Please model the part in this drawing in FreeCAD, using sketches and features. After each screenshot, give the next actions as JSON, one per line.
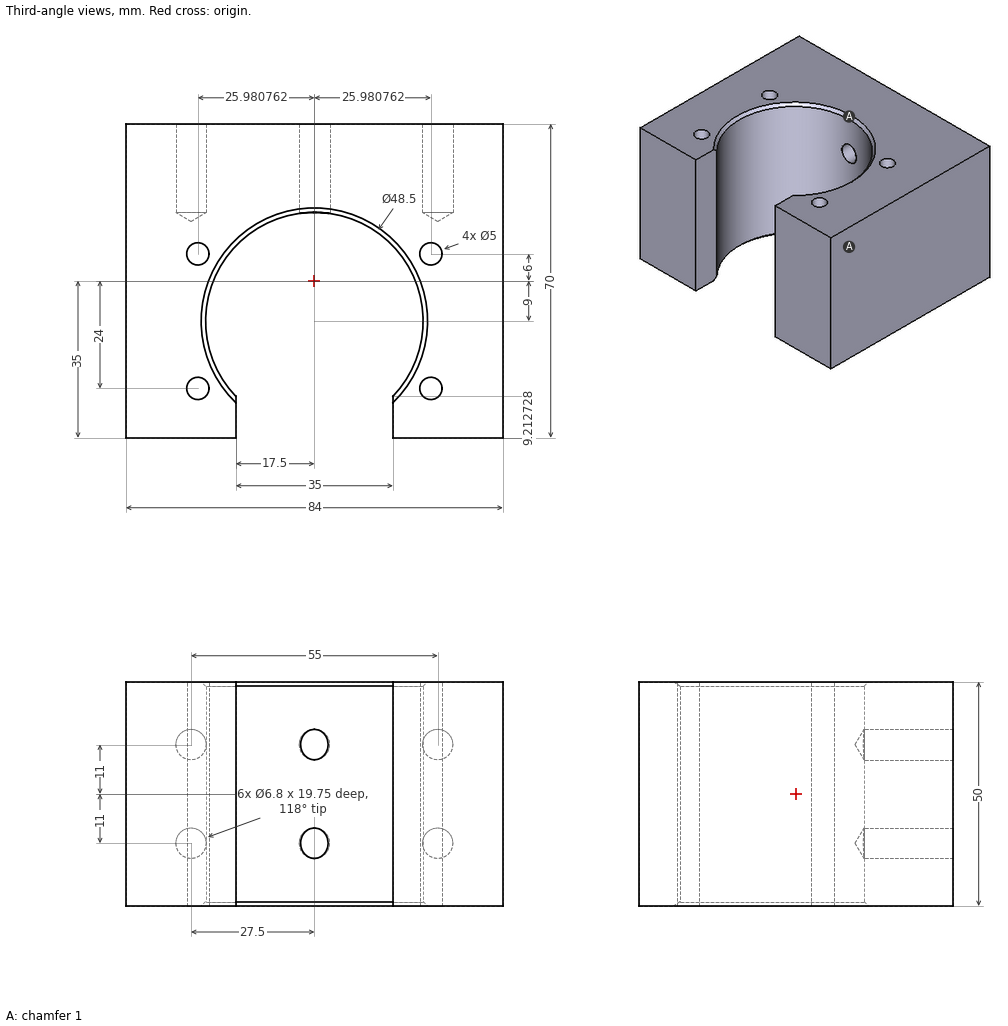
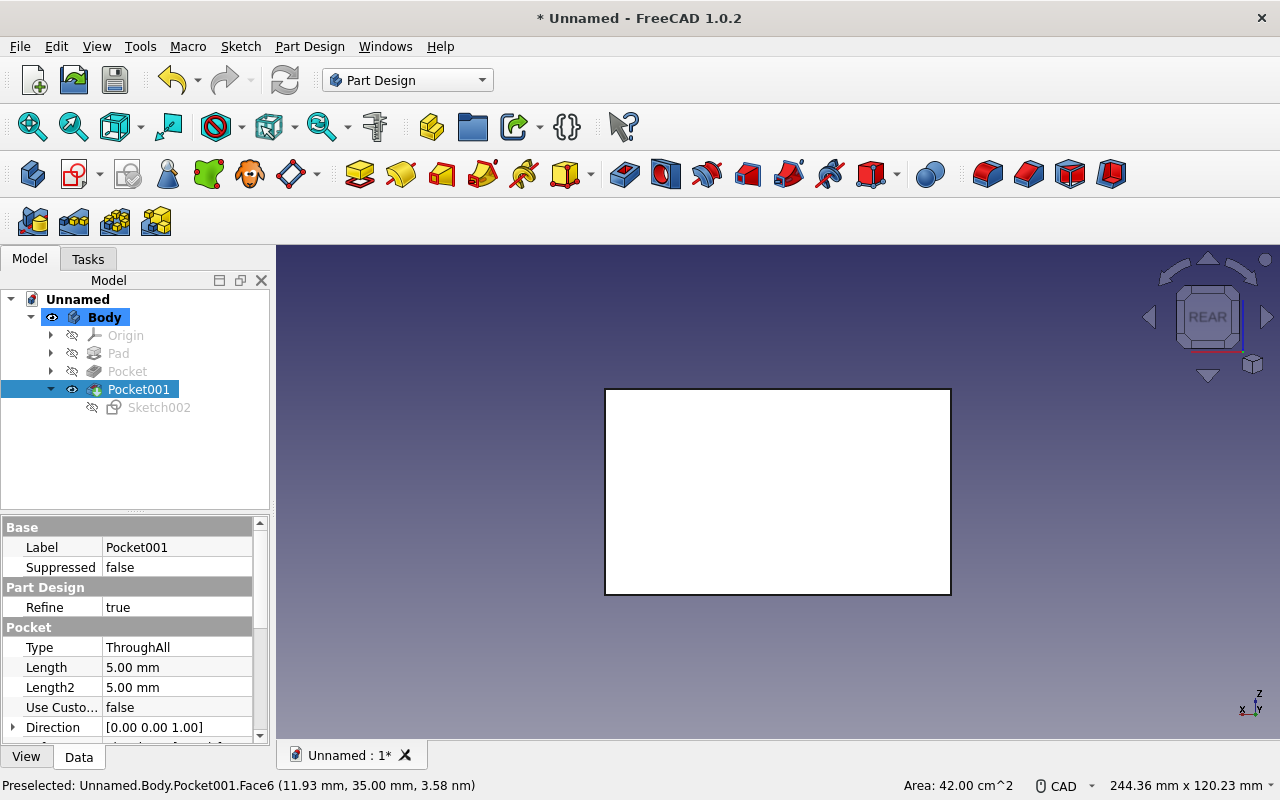
{"action": "left_click", "coordinate": [74, 174]}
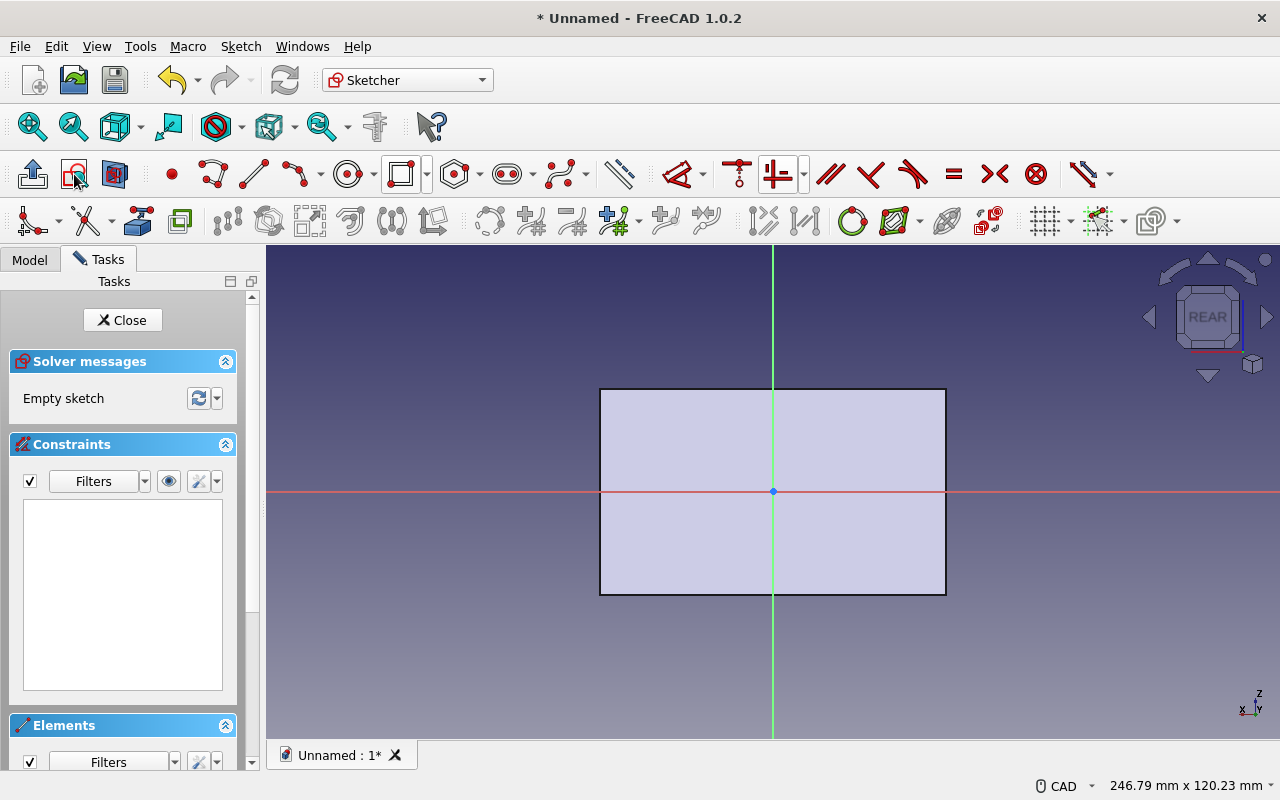
{"action": "scroll", "coordinate": [829, 492], "scroll_direction": "up", "scroll_amount": 4}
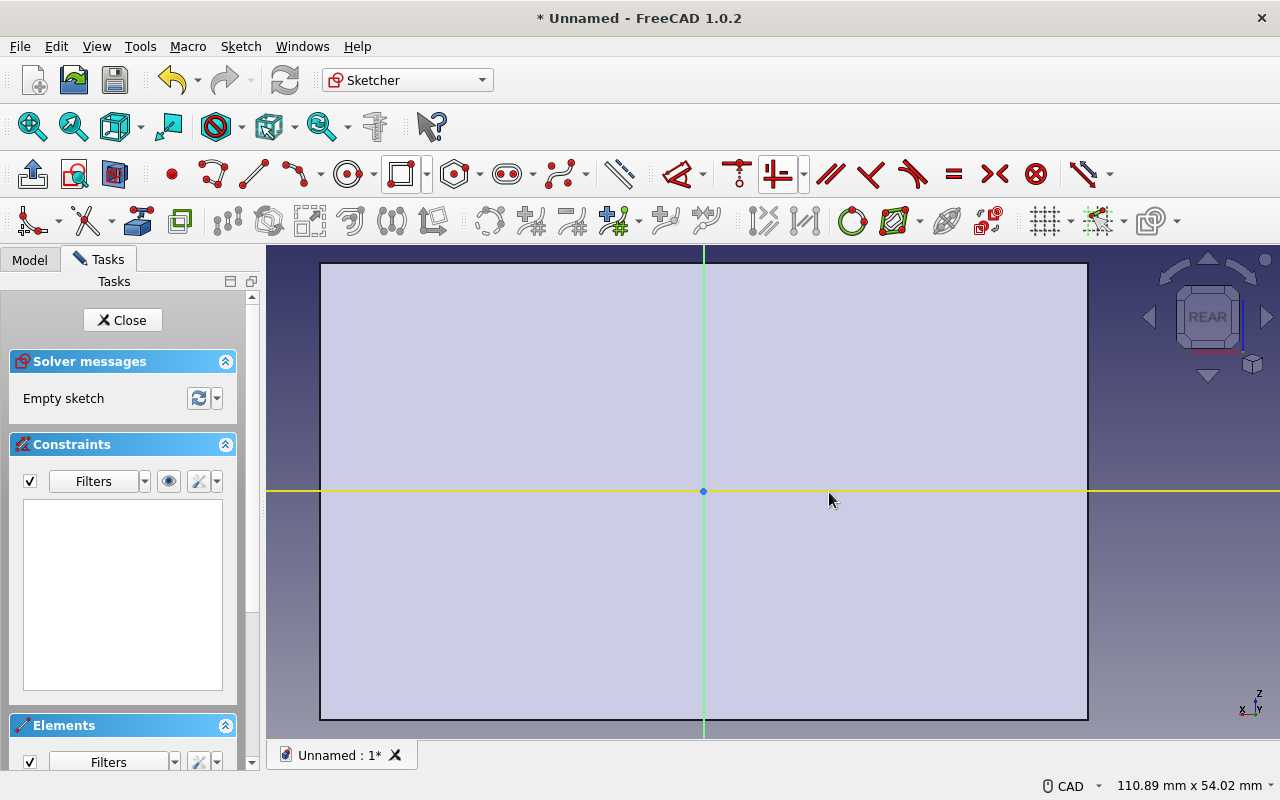
{"action": "left_click", "coordinate": [348, 174]}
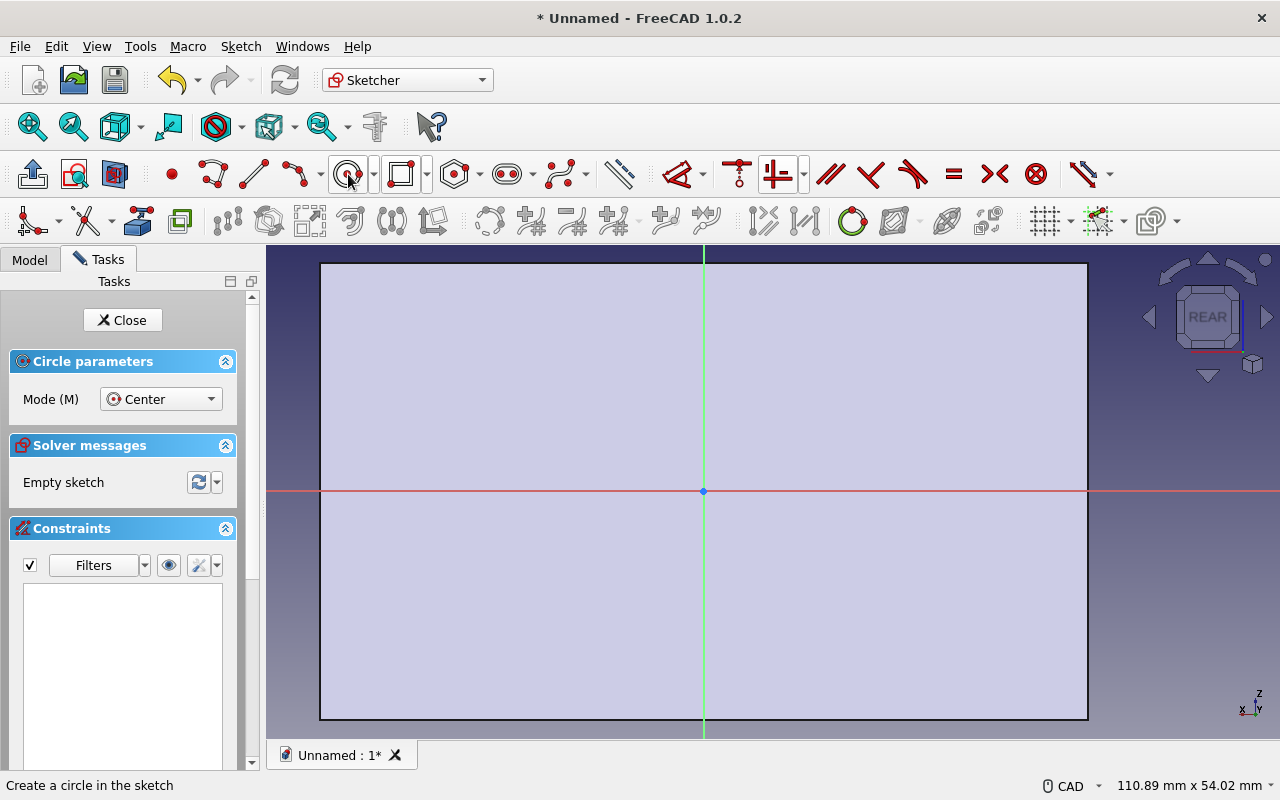
{"action": "left_click", "coordinate": [955, 592]}
{"action": "mouse_move", "coordinate": [977, 570]}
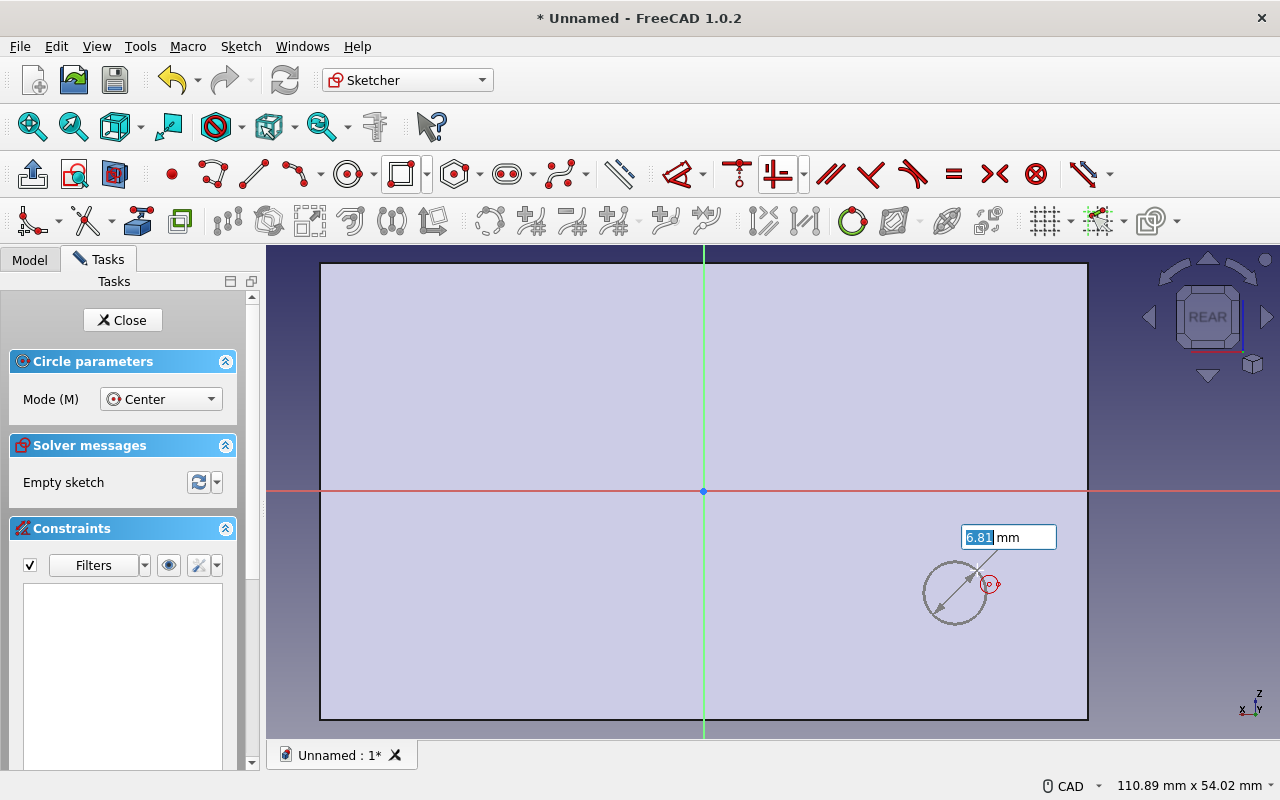
{"action": "type", "text": "6.8"}
{"action": "key", "text": "Return"}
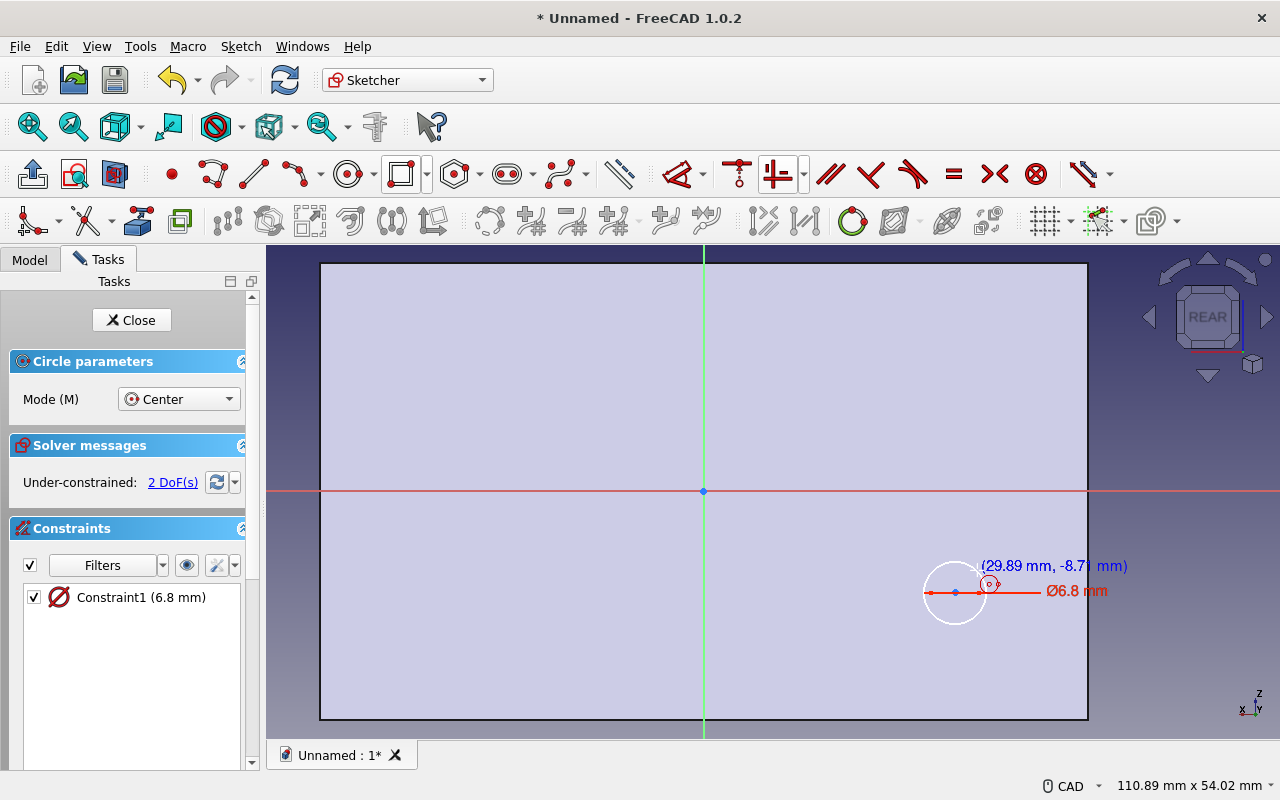
{"action": "left_click", "coordinate": [955, 391]}
{"action": "mouse_move", "coordinate": [977, 369]}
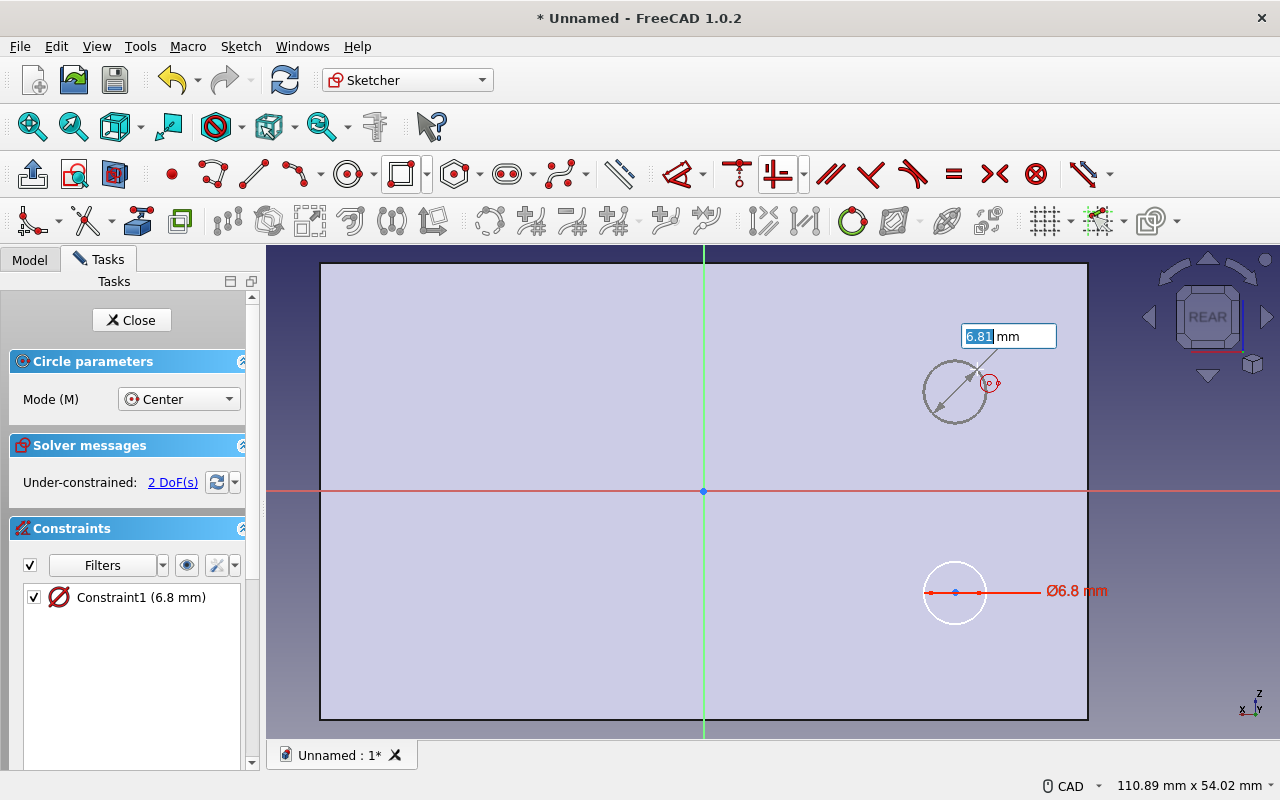
{"action": "type", "text": "6.8"}
{"action": "key", "text": "Return"}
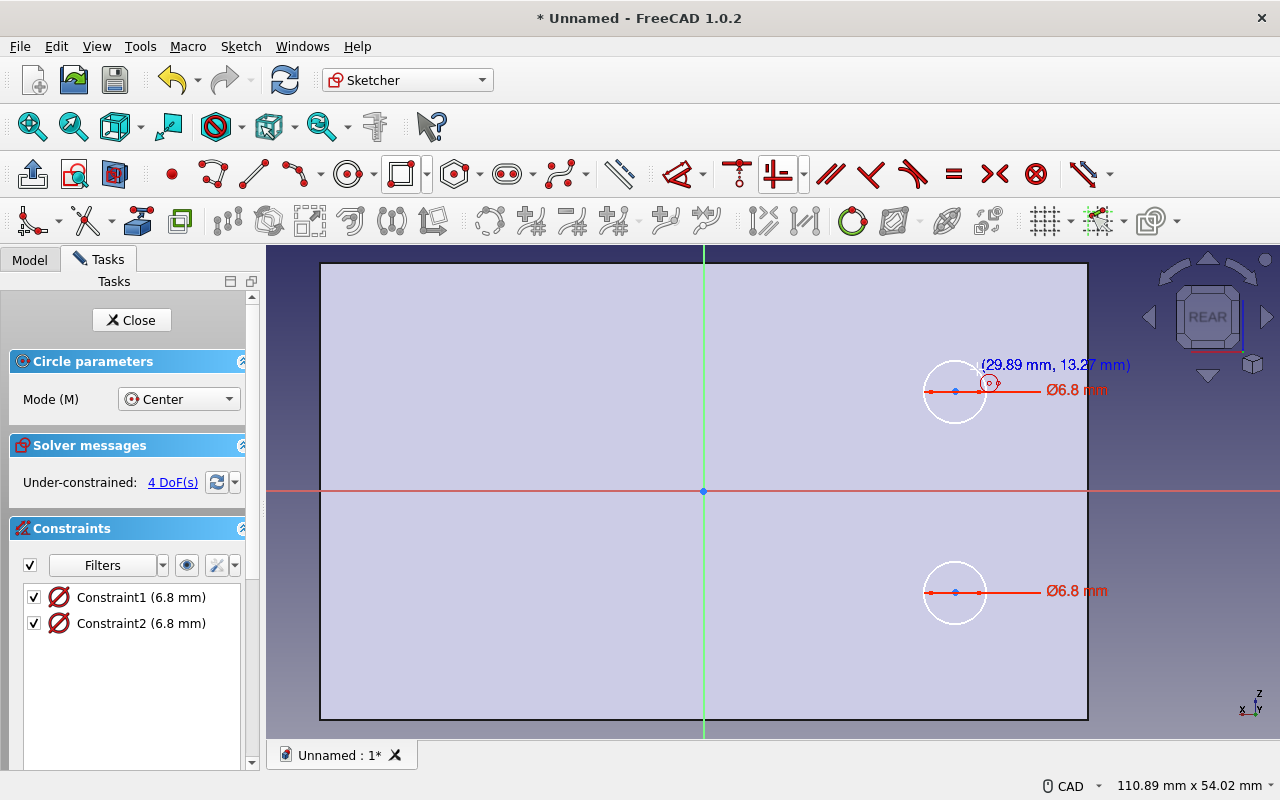
{"action": "left_click", "coordinate": [452, 391]}
{"action": "mouse_move", "coordinate": [474, 369]}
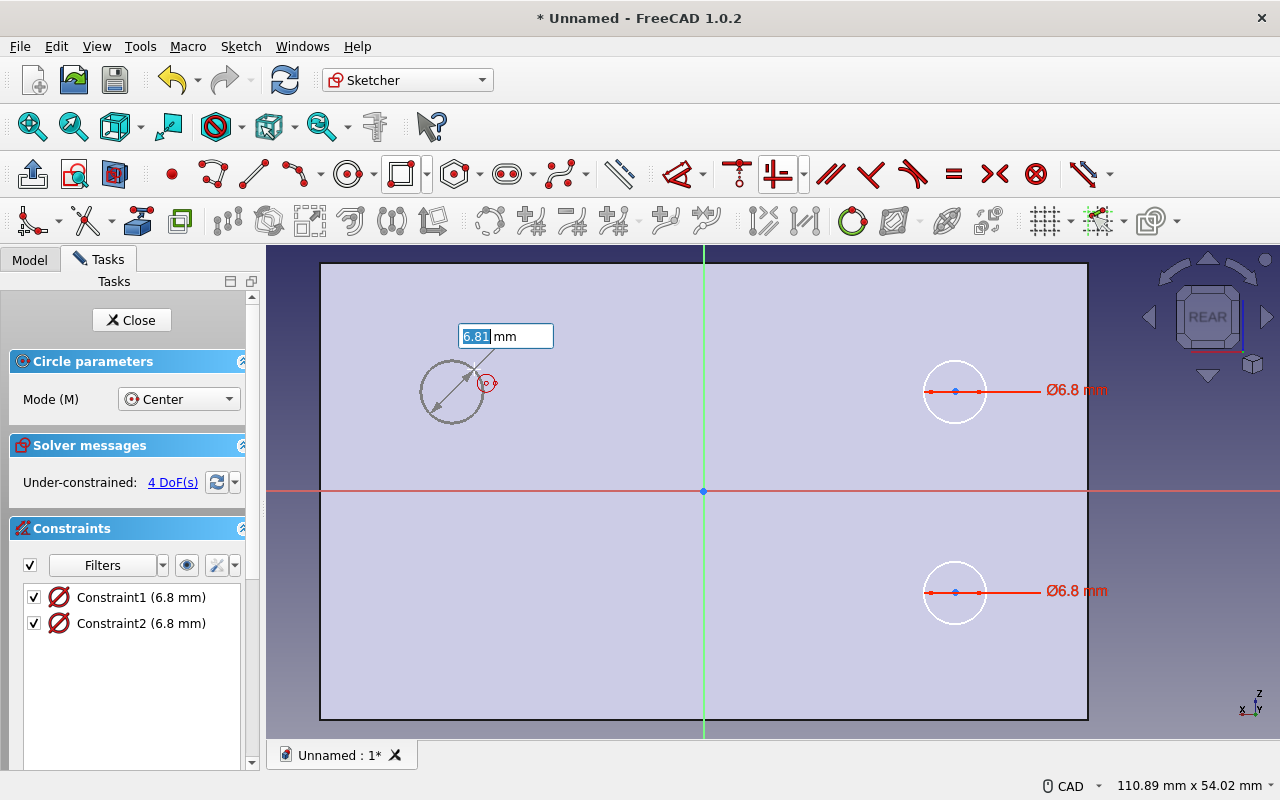
{"action": "type", "text": "6.8"}
{"action": "key", "text": "Return"}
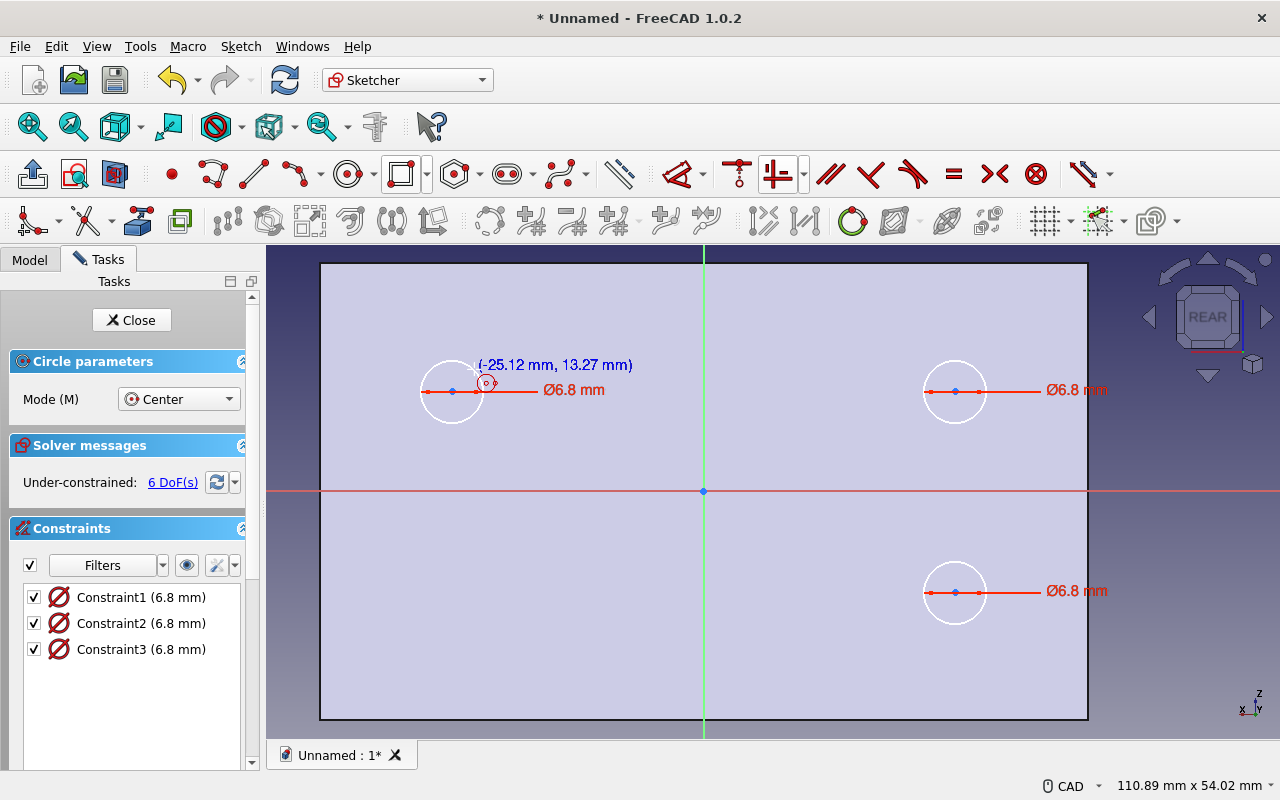
{"action": "left_click", "coordinate": [452, 592]}
{"action": "mouse_move", "coordinate": [474, 570]}